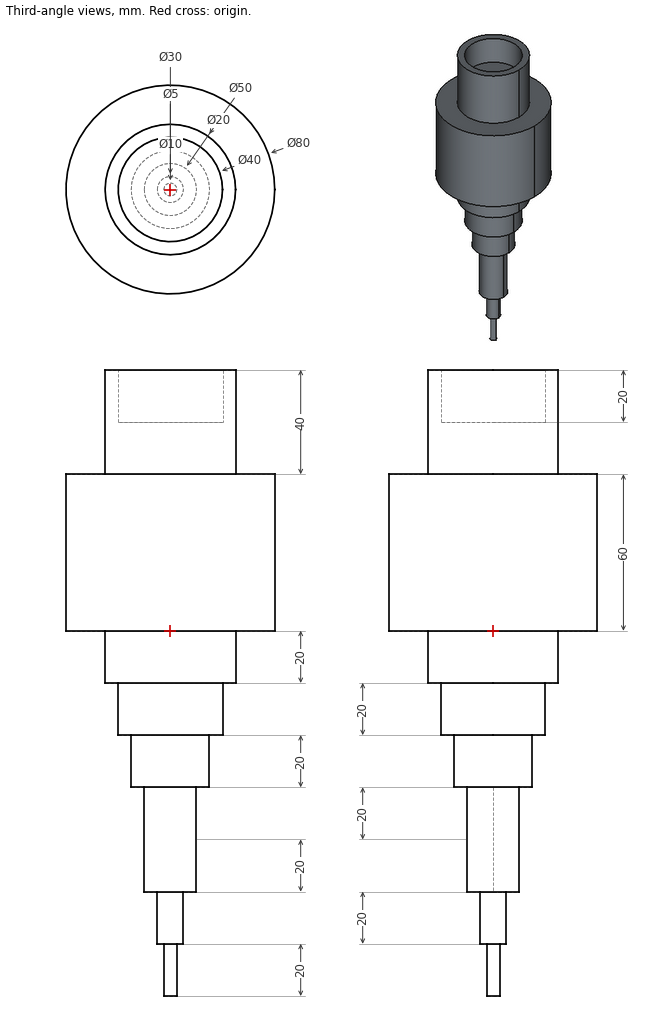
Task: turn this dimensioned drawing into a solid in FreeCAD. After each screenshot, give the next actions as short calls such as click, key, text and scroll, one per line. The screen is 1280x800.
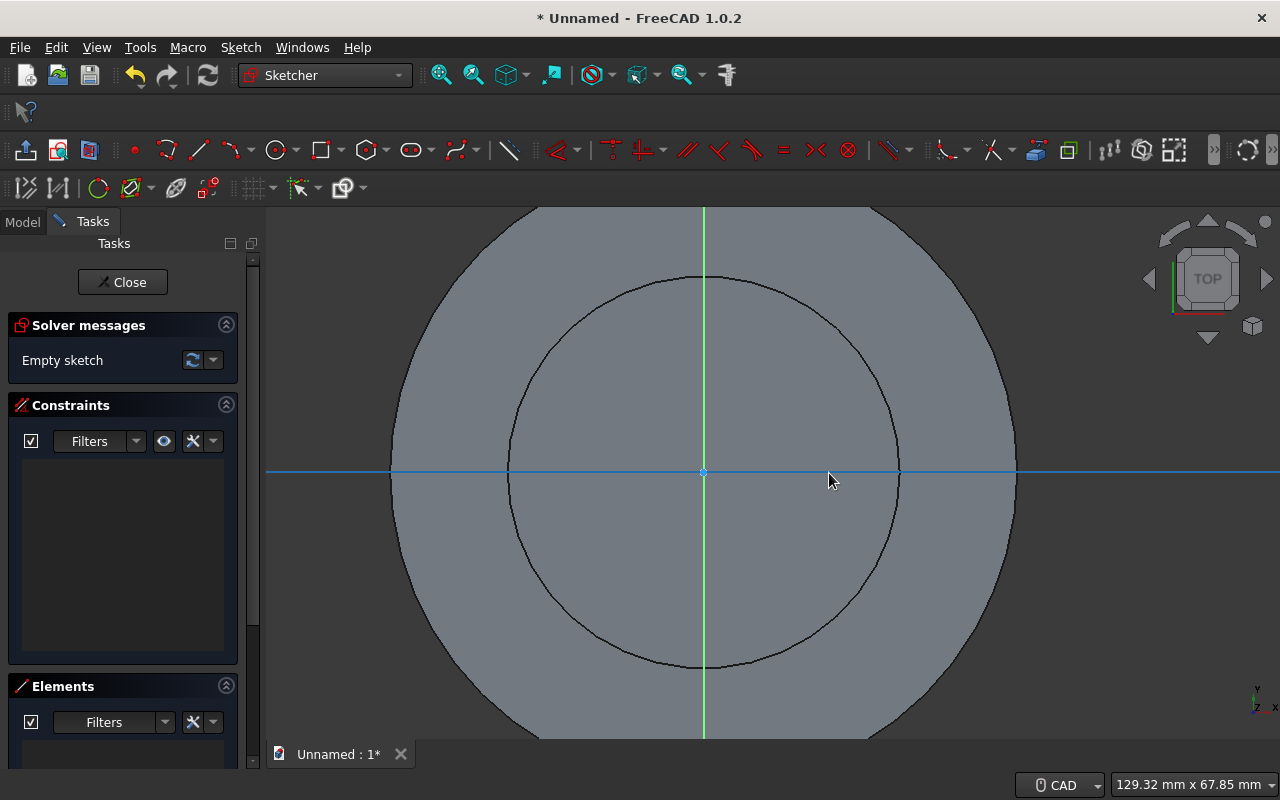
click(276, 150)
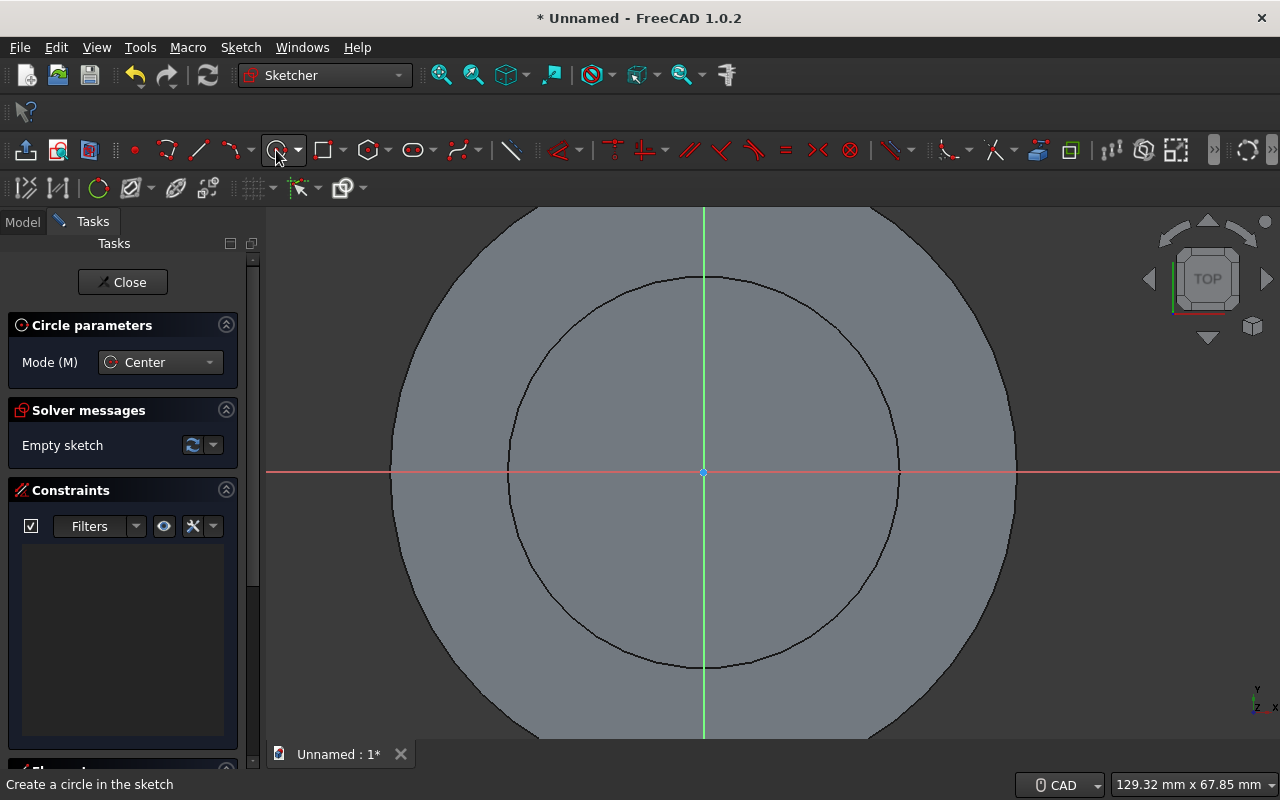
click(704, 472)
click(815, 361)
key(Escape)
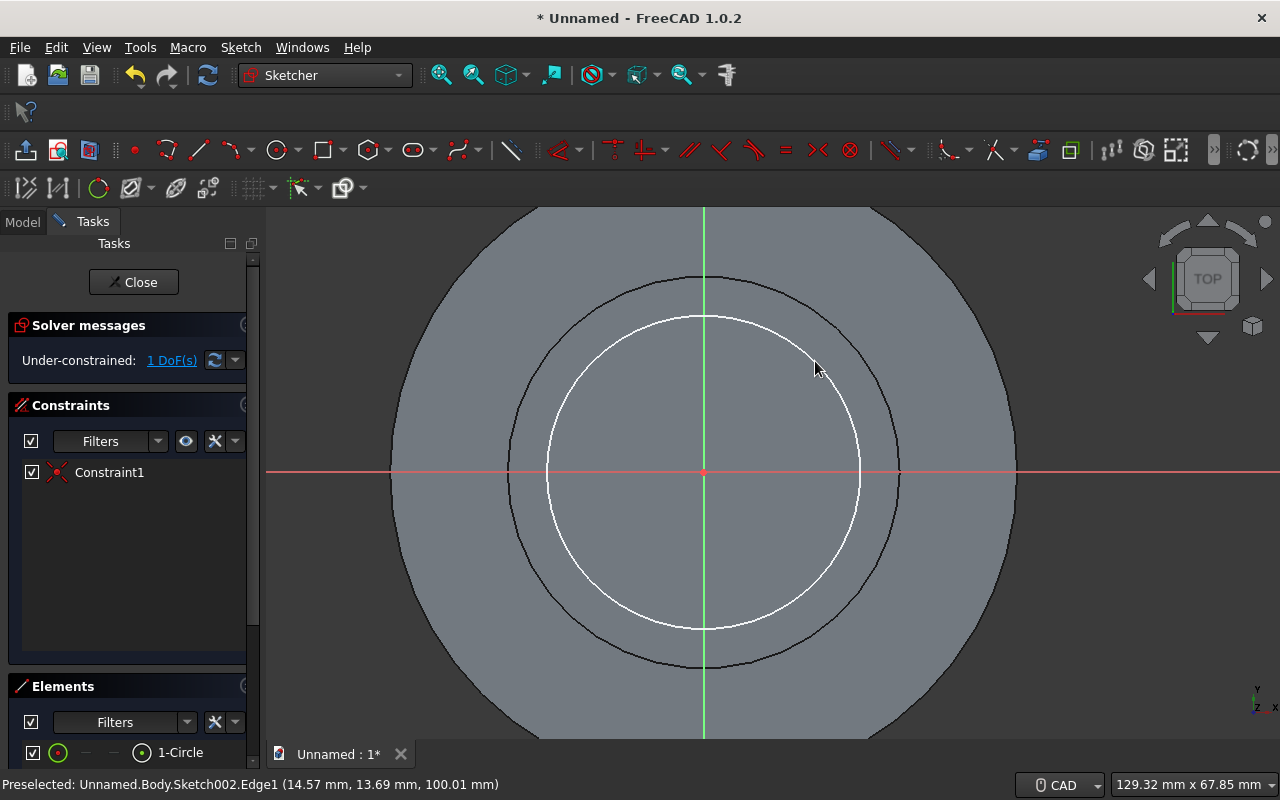
click(558, 150)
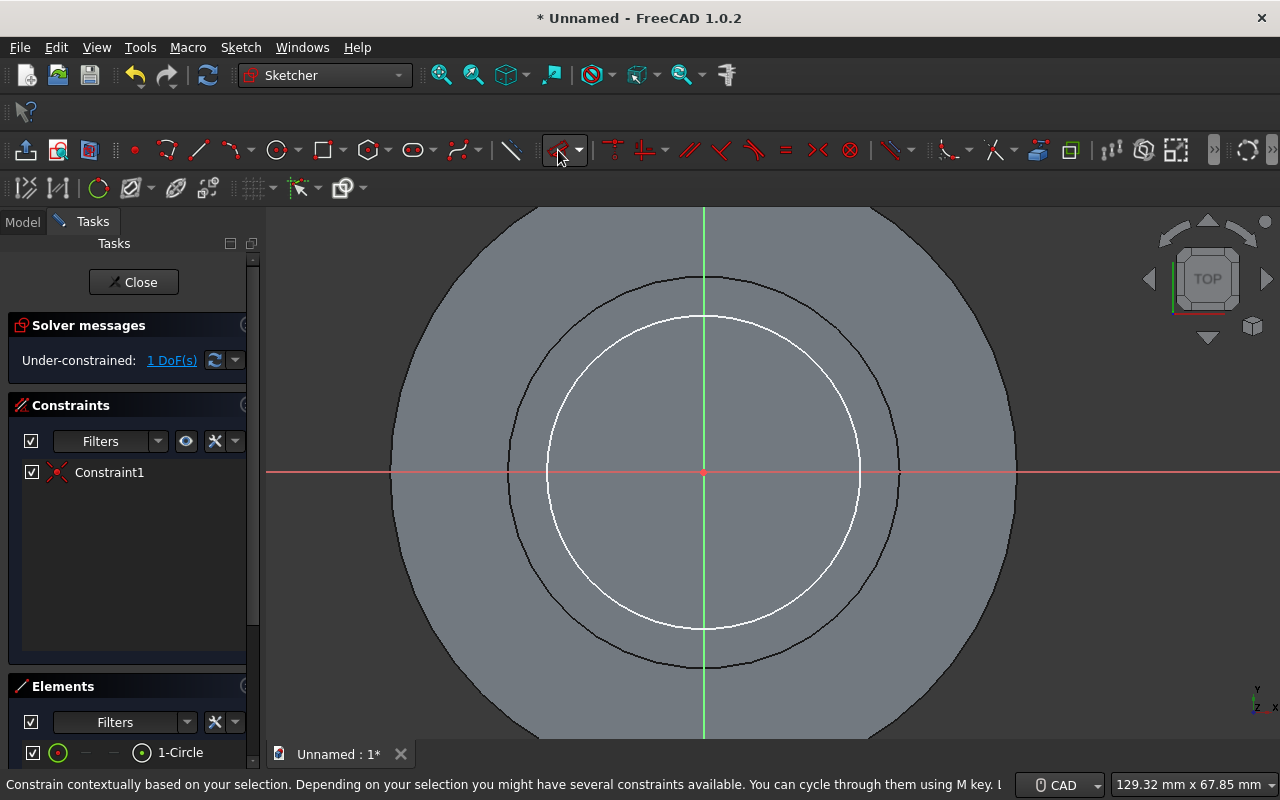
click(814, 361)
click(837, 338)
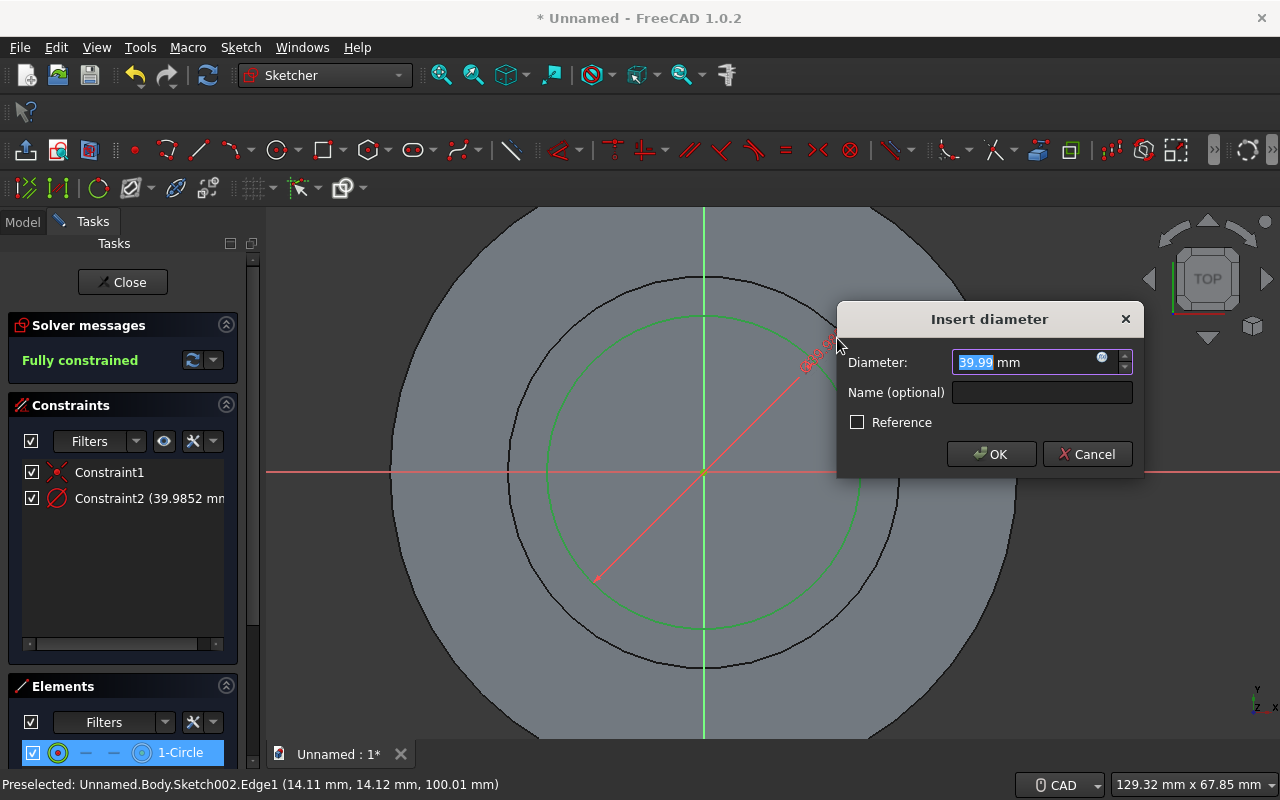
text(40)
key(Return)
key(Escape)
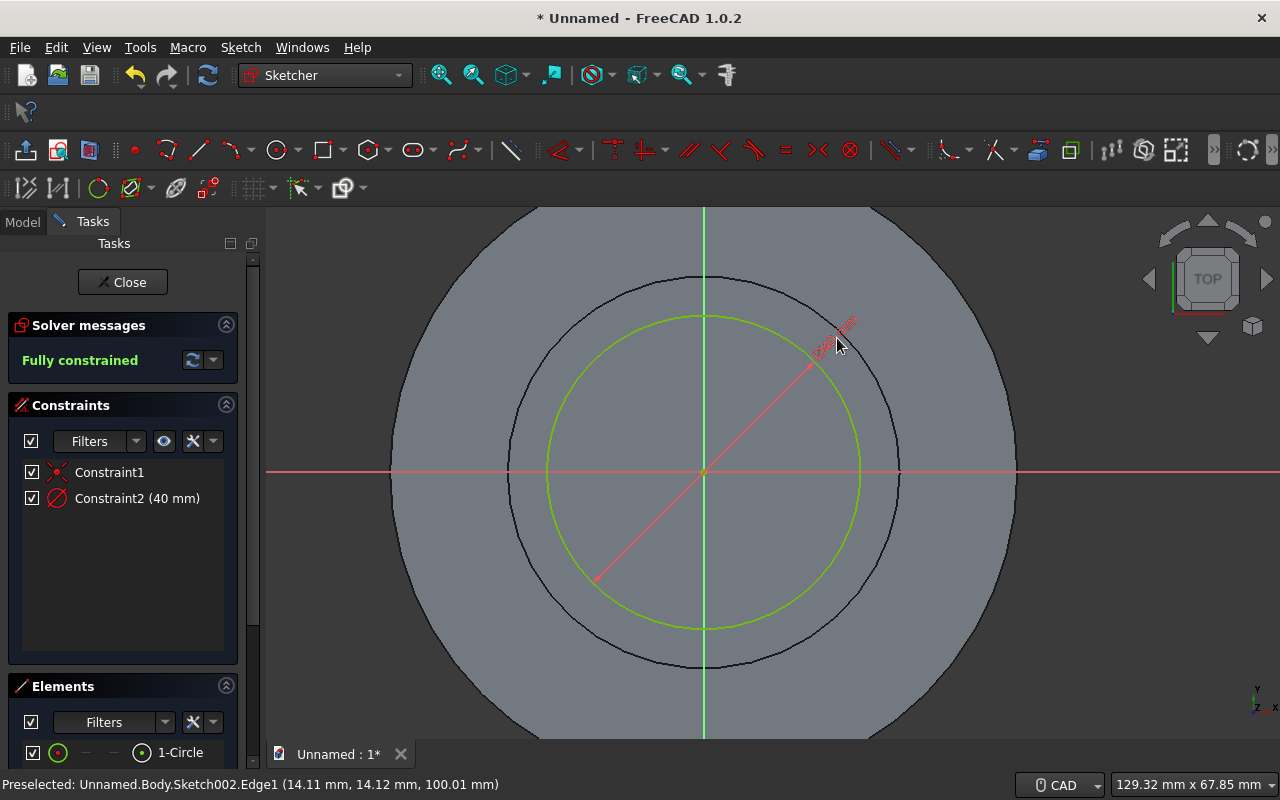
click(123, 282)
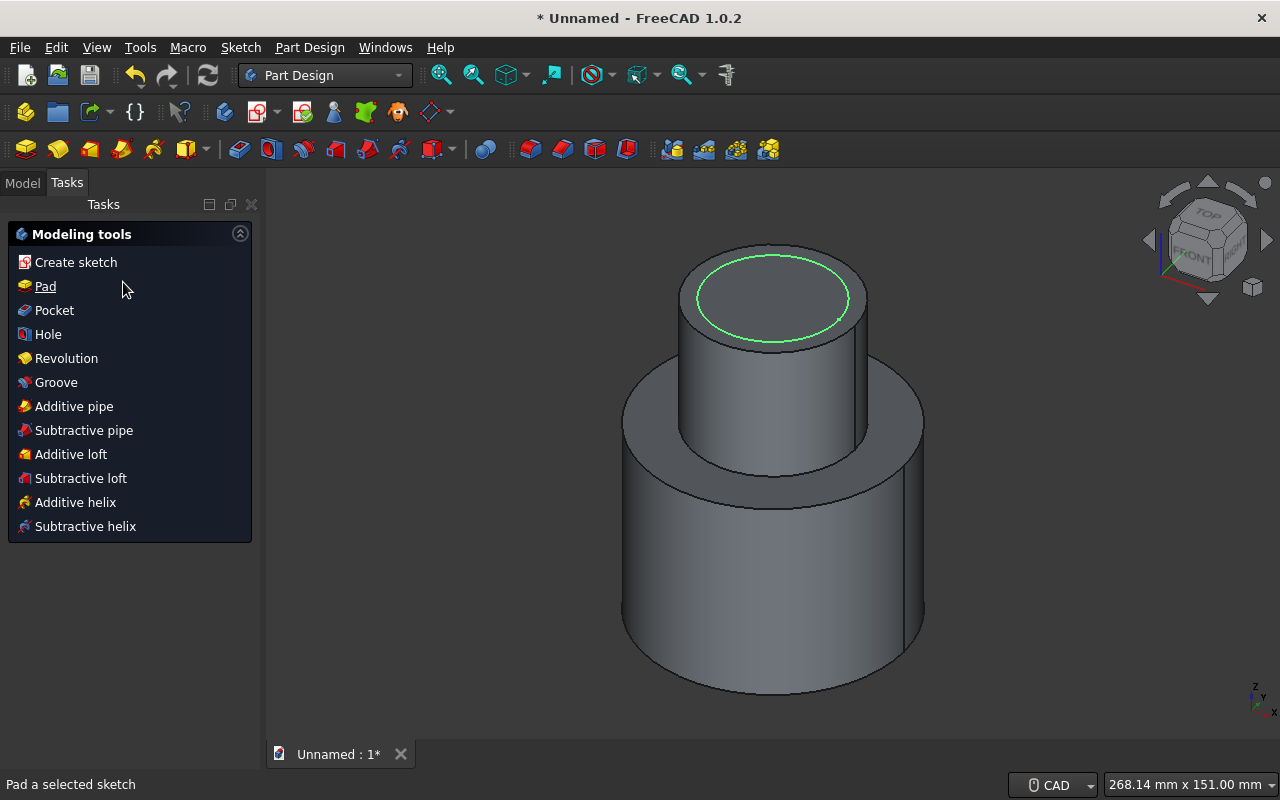
click(240, 150)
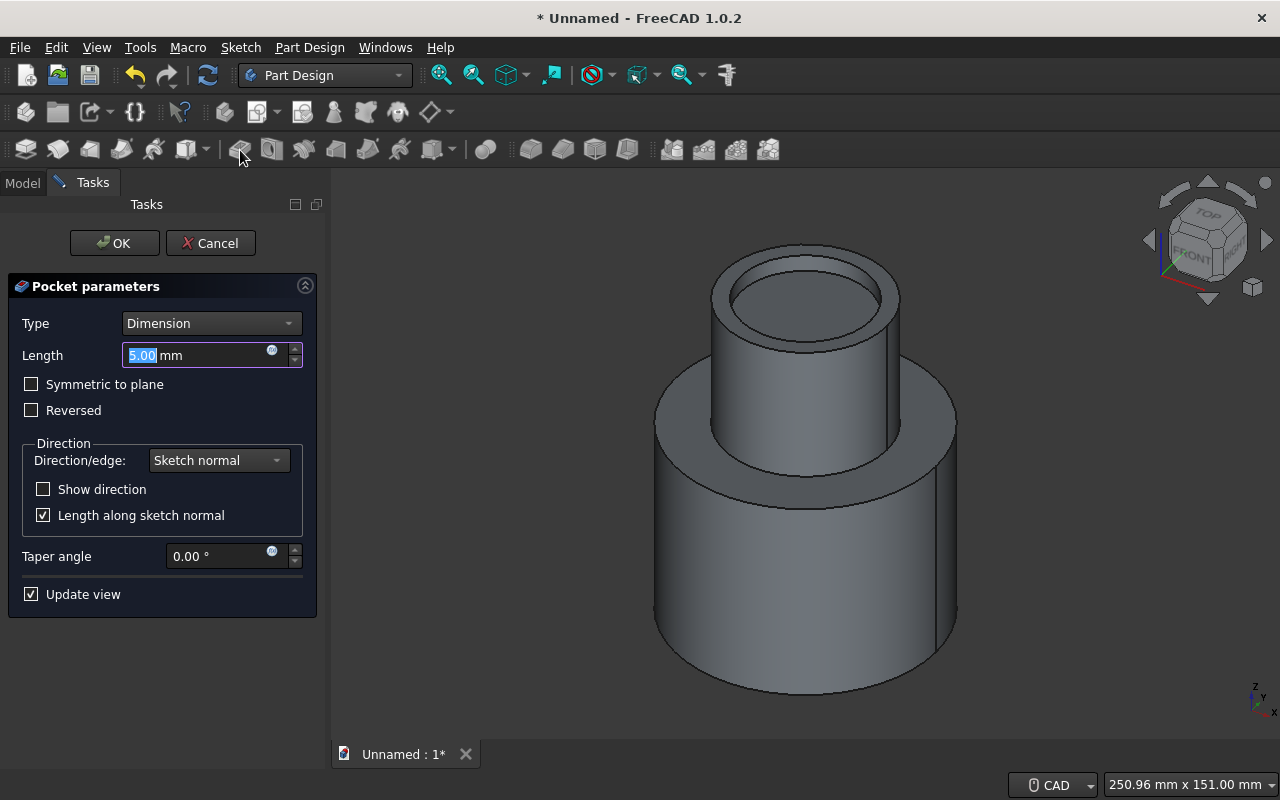
text(20)
key(Tab)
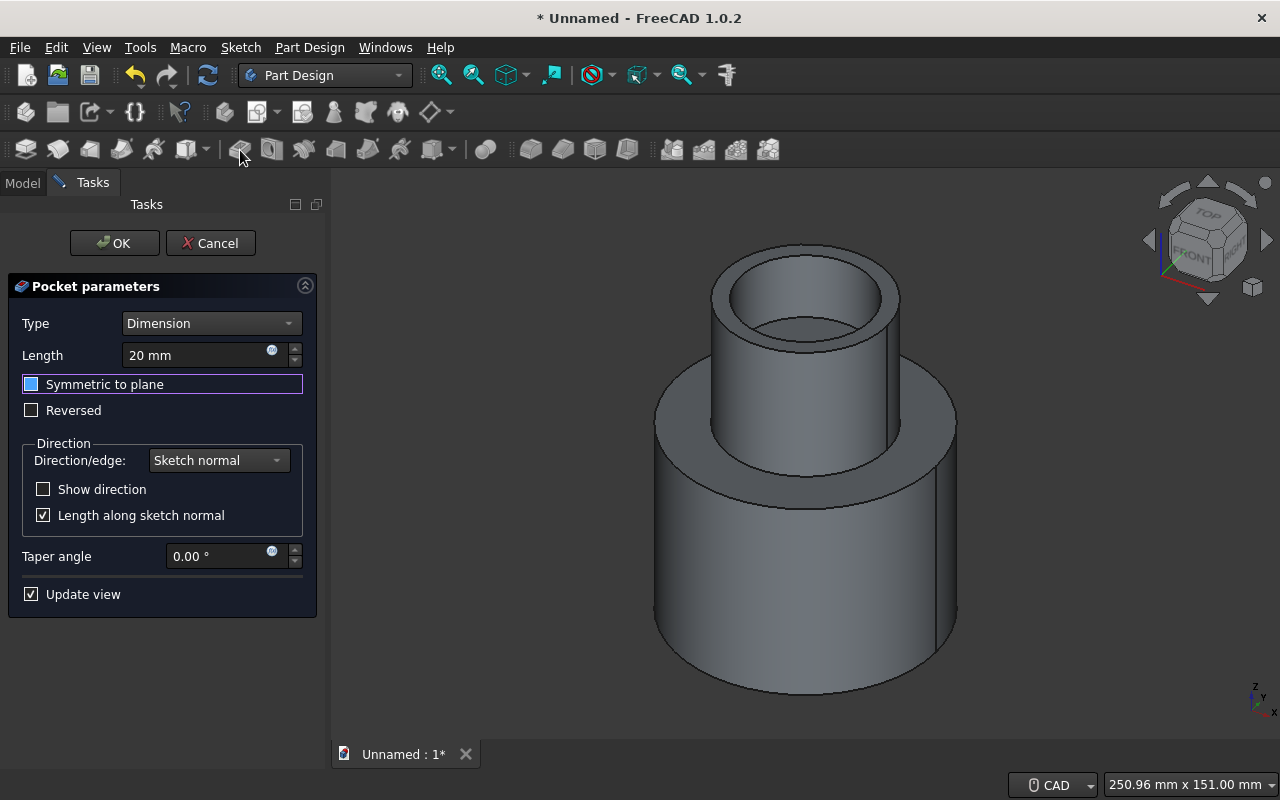
click(115, 243)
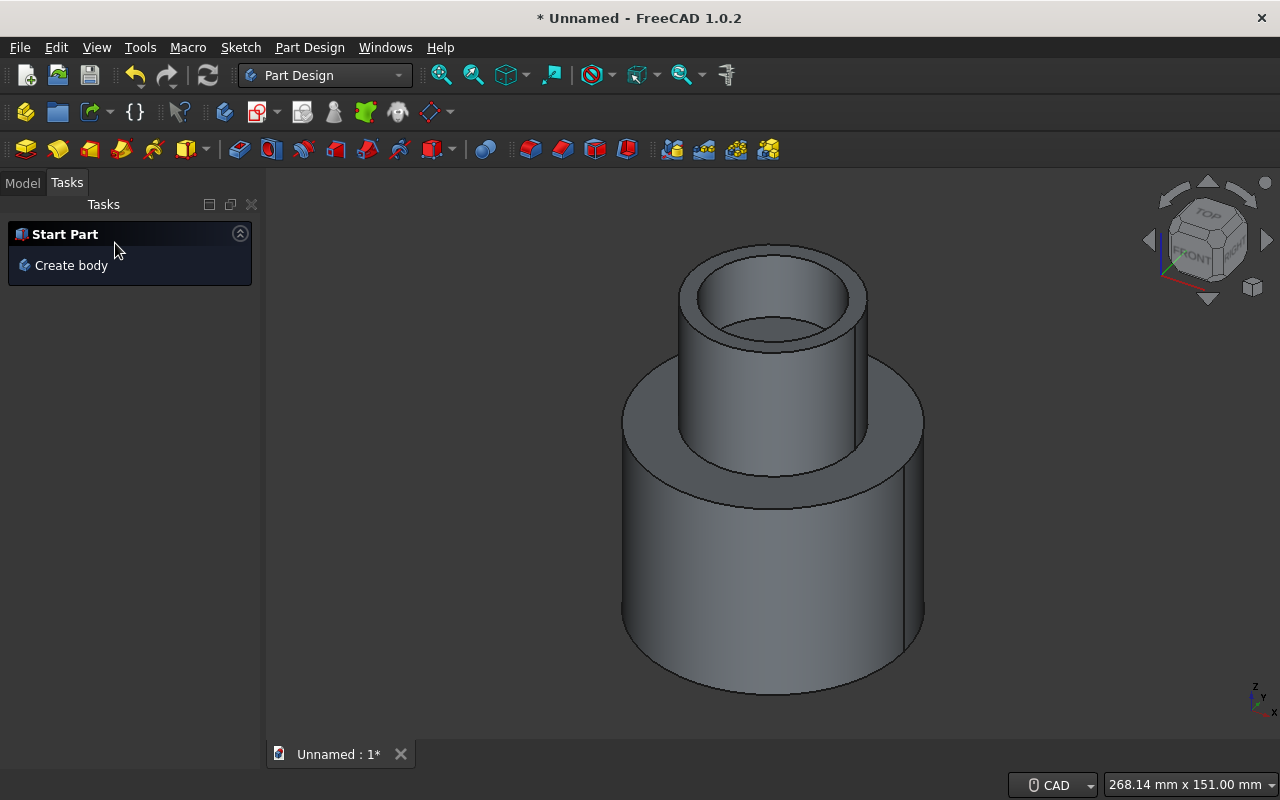
click(23, 182)